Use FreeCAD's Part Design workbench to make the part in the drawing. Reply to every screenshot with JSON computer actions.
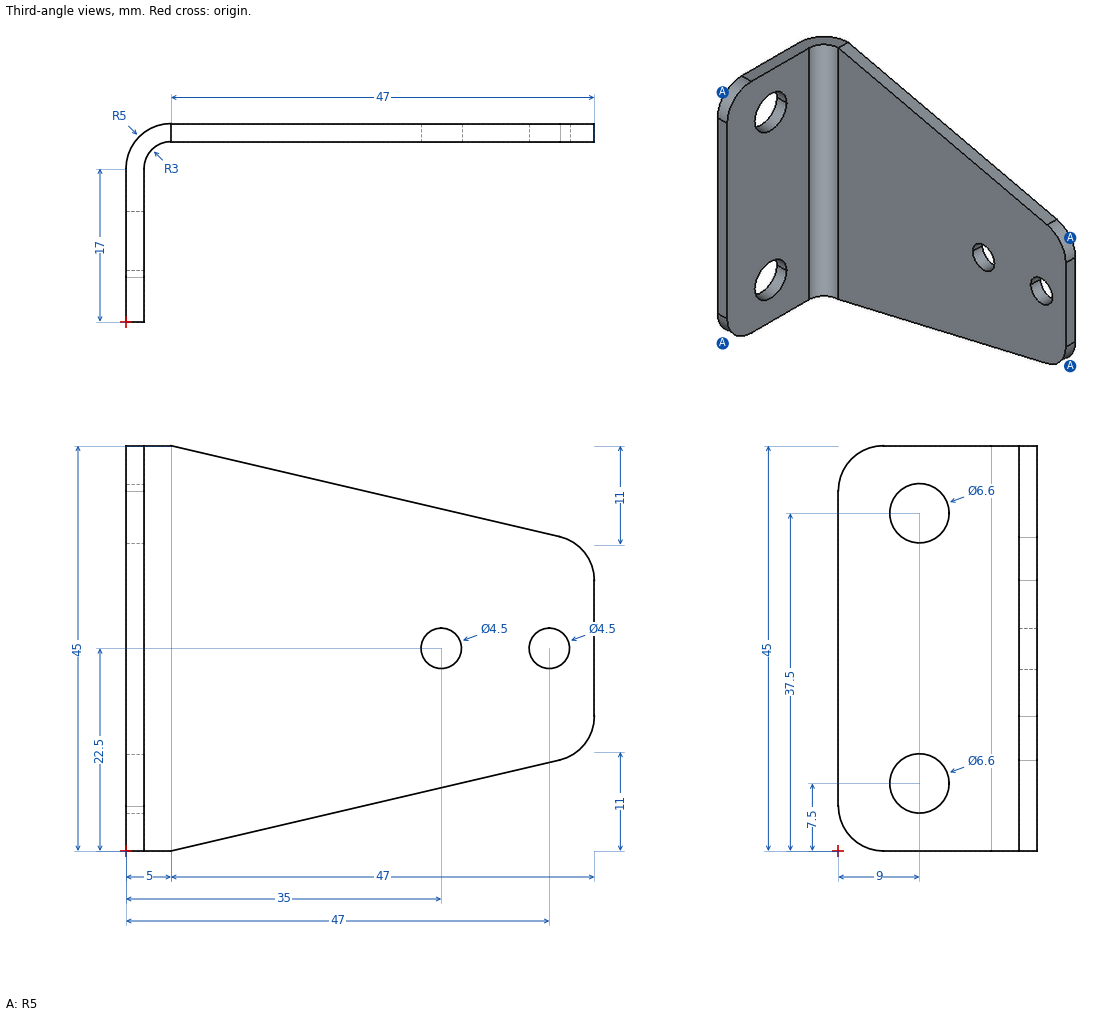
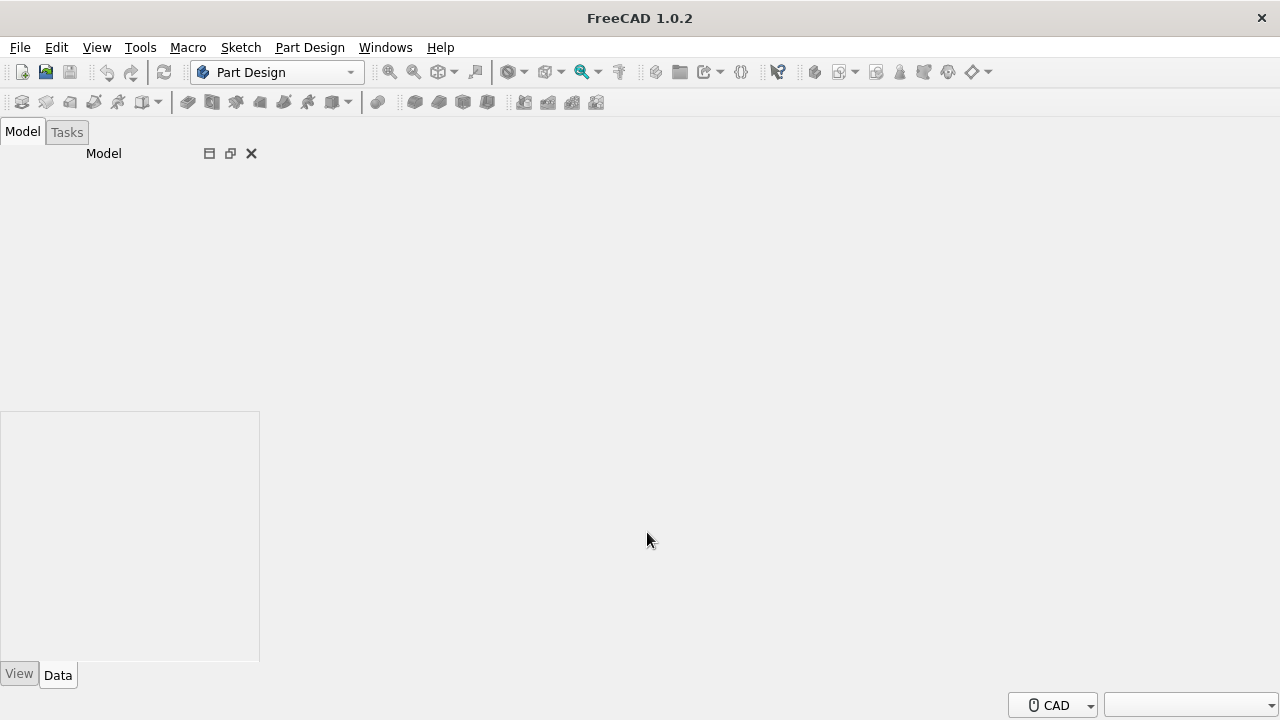
{"action": "key", "text": "ctrl+n"}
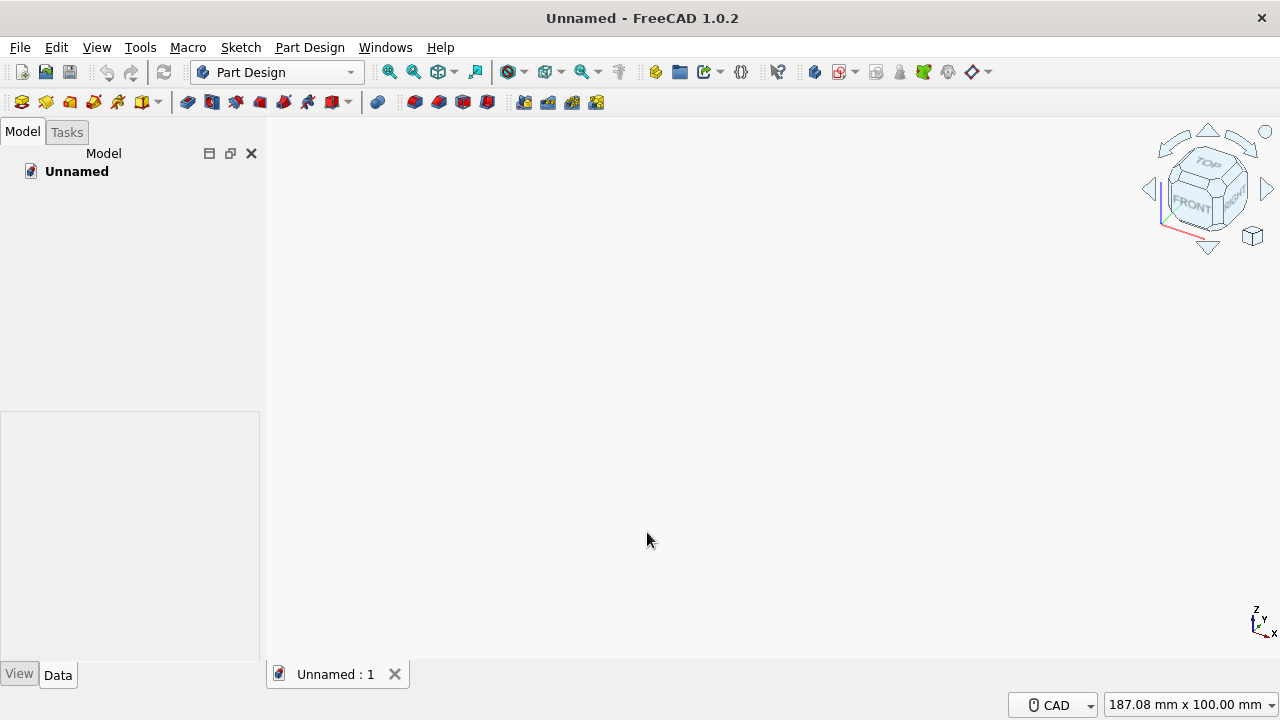
{"action": "left_click", "coordinate": [840, 72]}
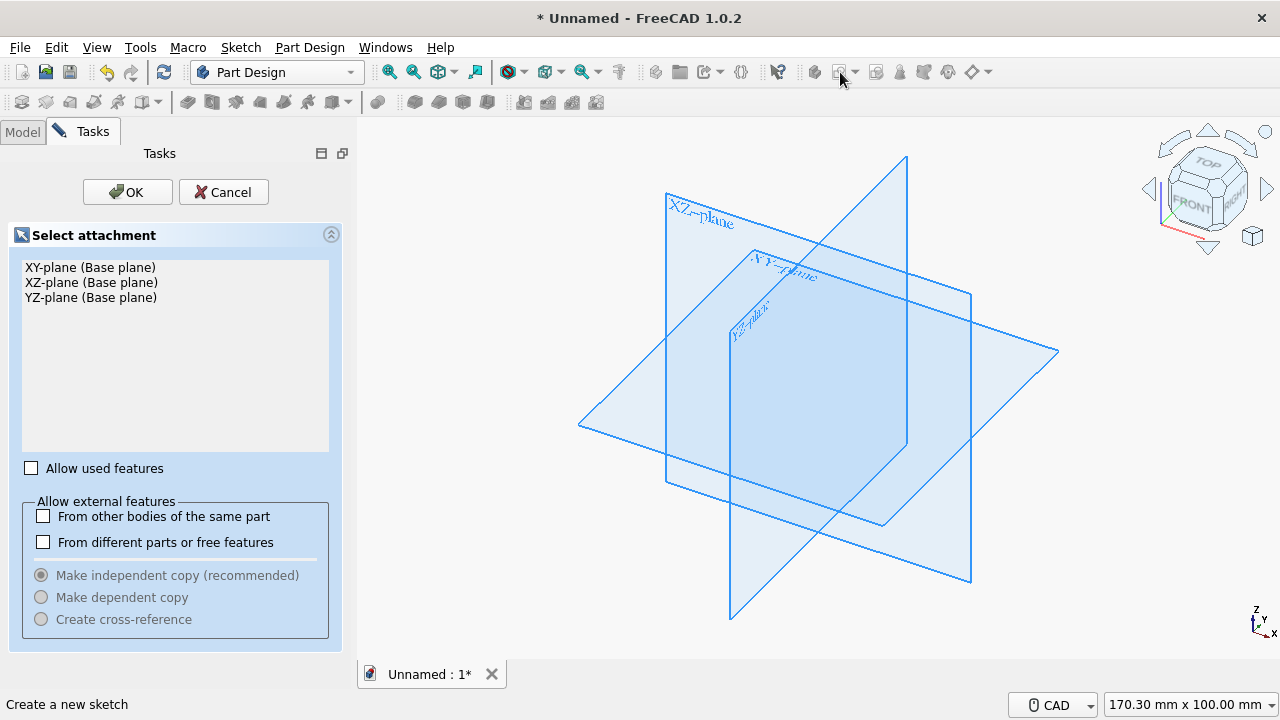
{"action": "left_click", "coordinate": [82, 268]}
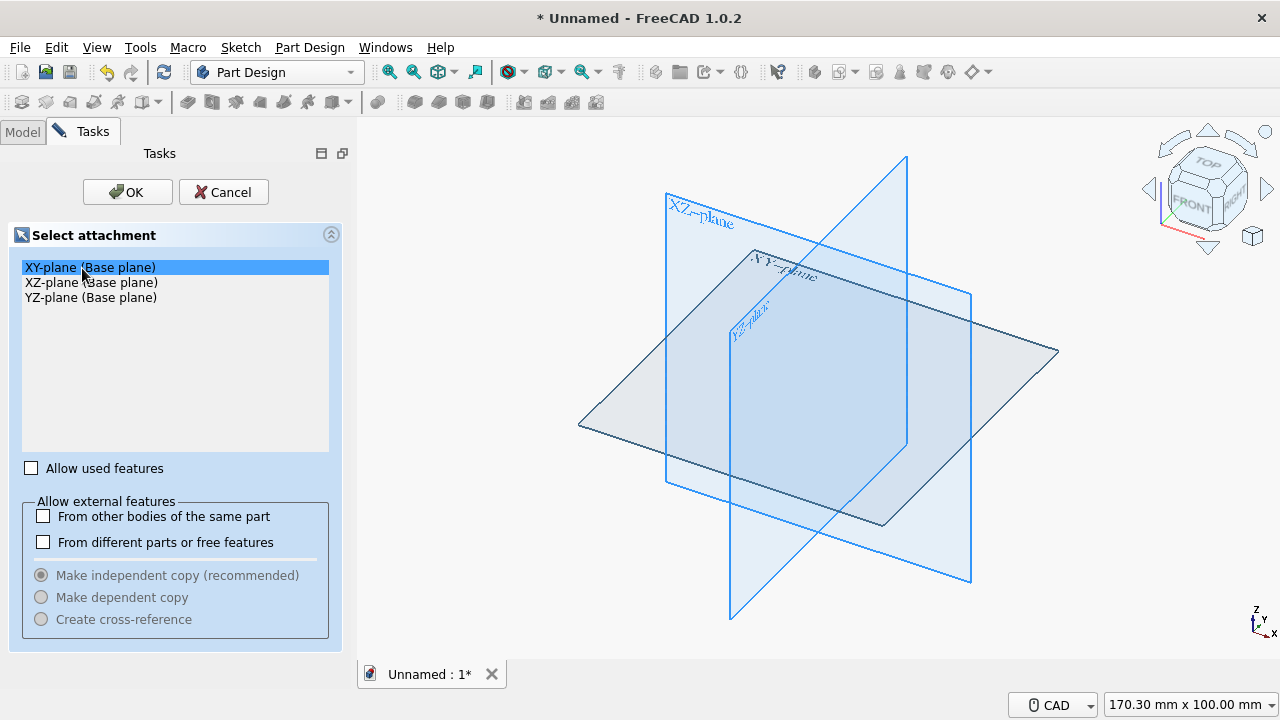
{"action": "left_click", "coordinate": [128, 192]}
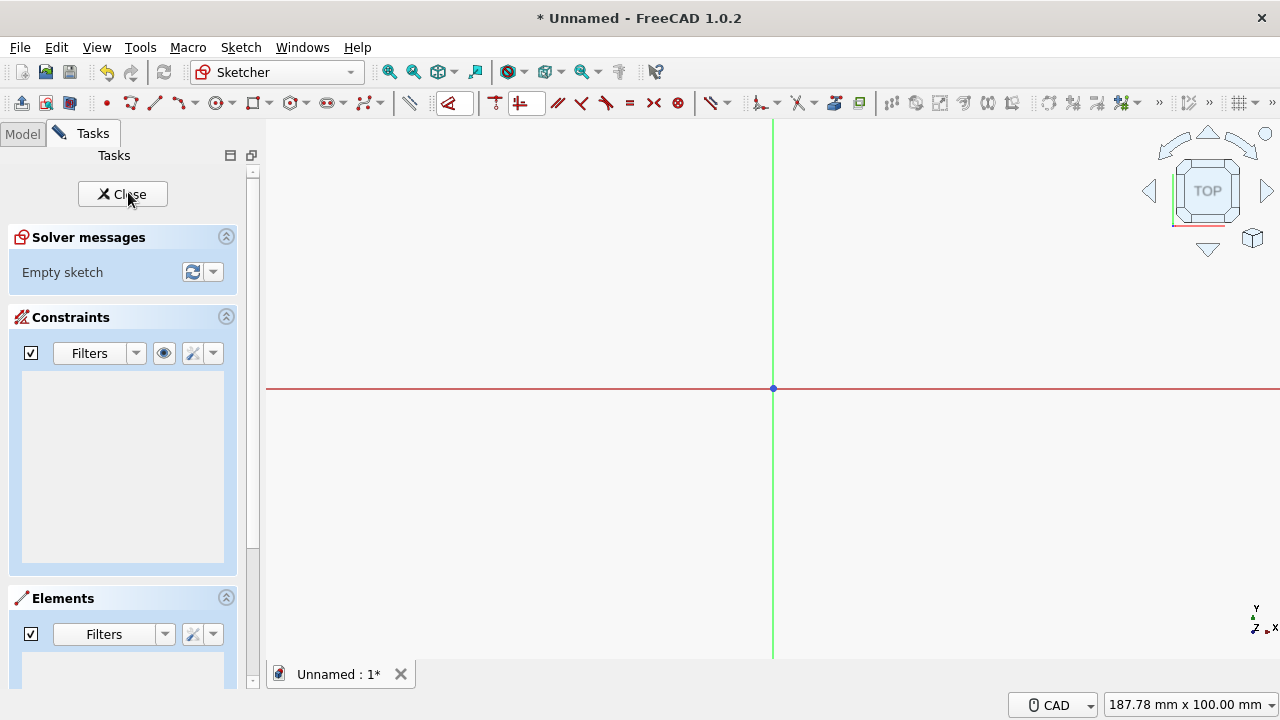
{"action": "scroll", "coordinate": [1084, 281], "scroll_direction": "up", "scroll_amount": 4}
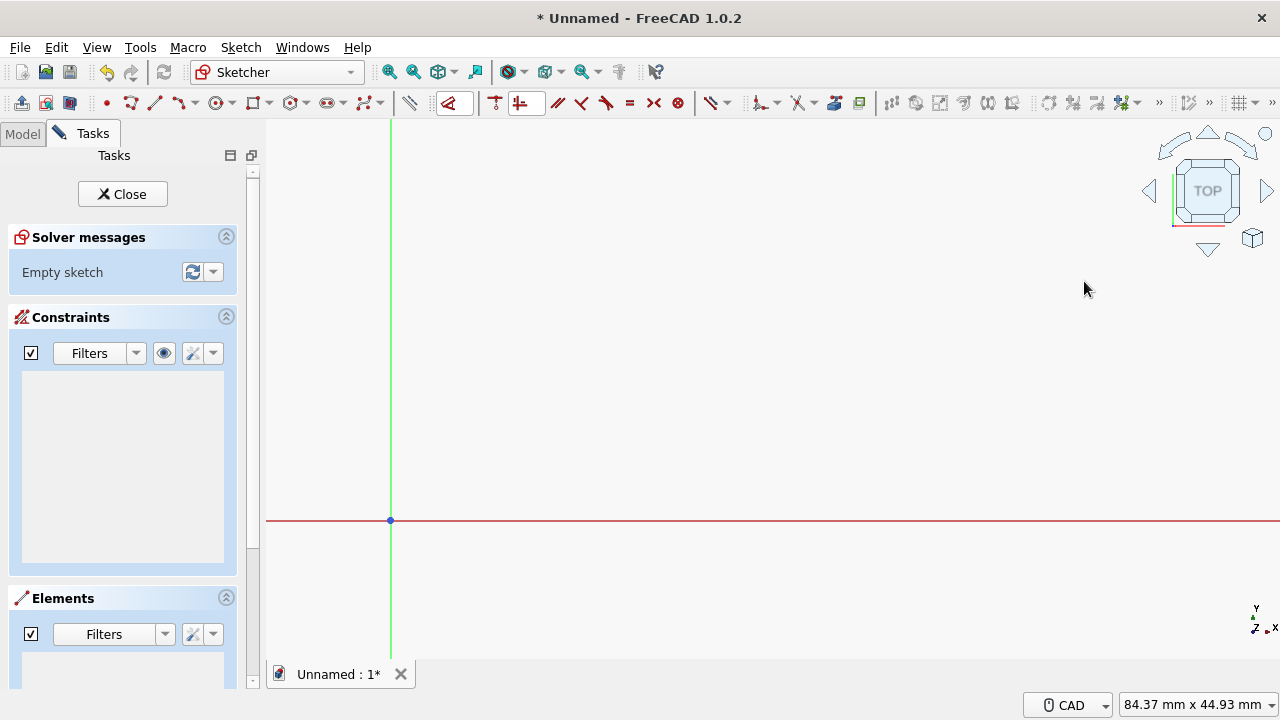
{"action": "left_click", "coordinate": [132, 104]}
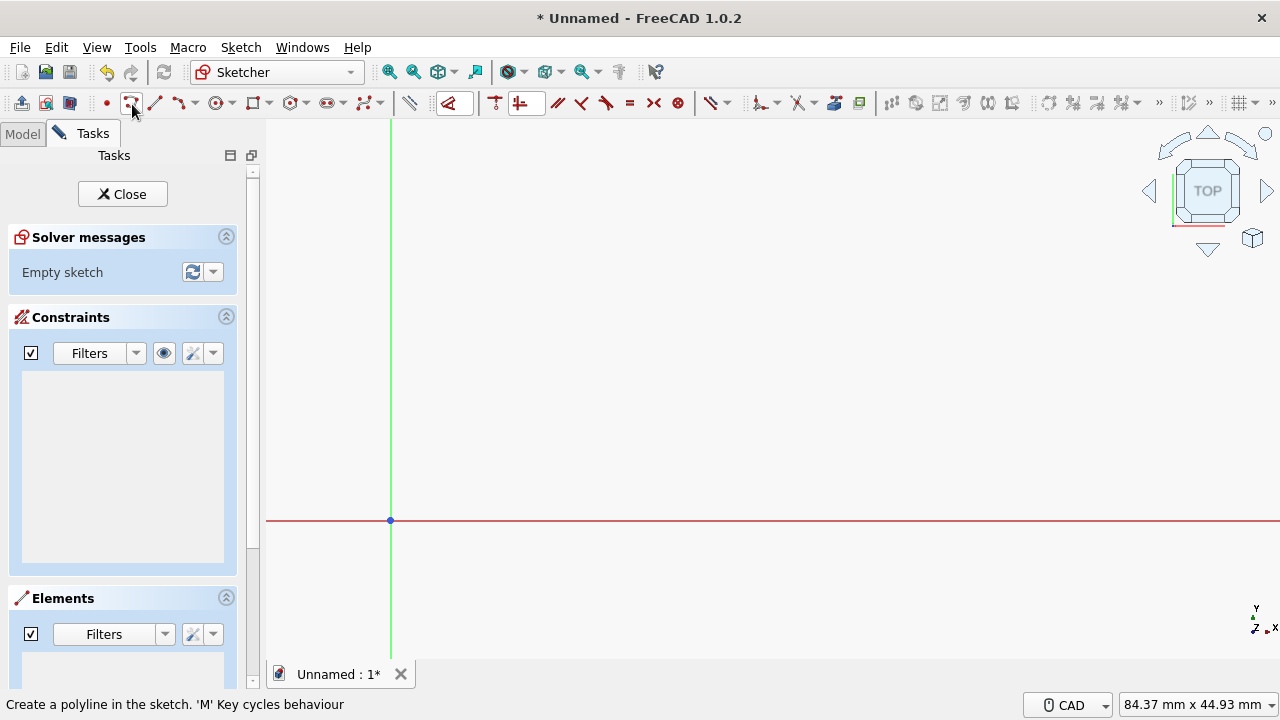
{"action": "left_click", "coordinate": [391, 317]}
{"action": "left_click", "coordinate": [391, 521]}
{"action": "left_click", "coordinate": [415, 512]}
{"action": "left_click", "coordinate": [415, 317]}
{"action": "right_click", "coordinate": [415, 317]}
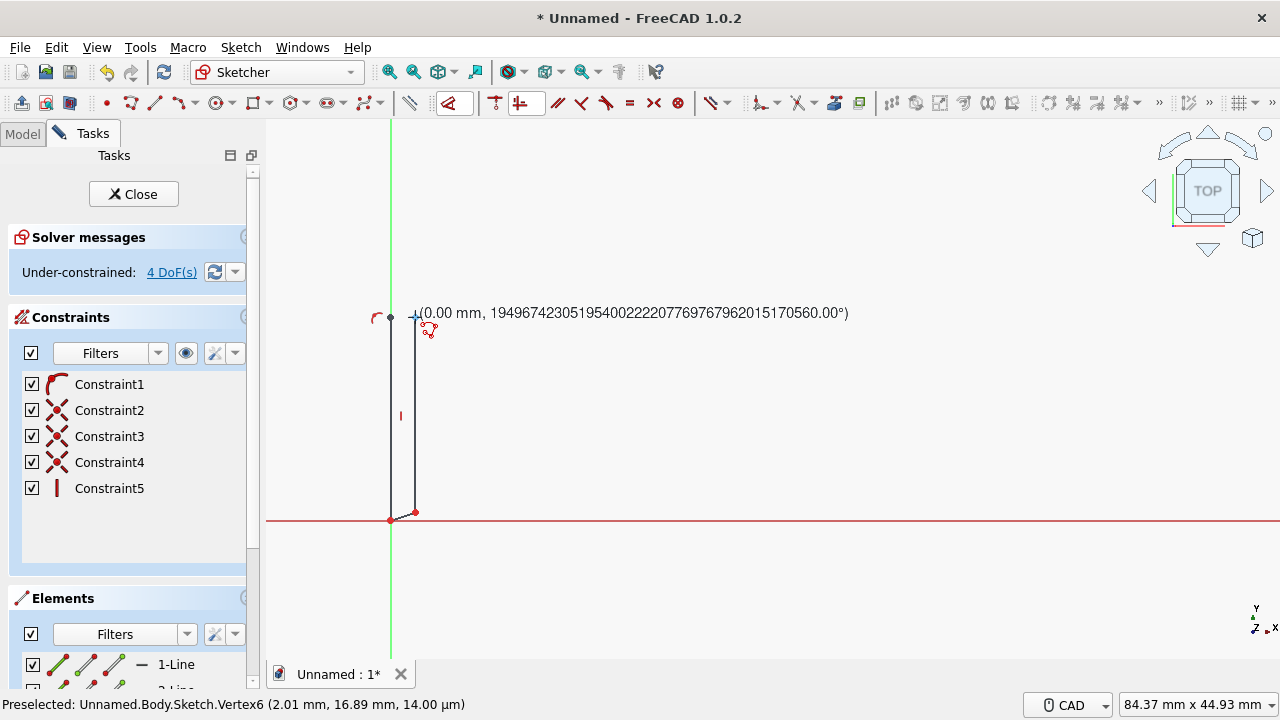
{"action": "left_click", "coordinate": [451, 281]}
{"action": "left_click", "coordinate": [1016, 281]}
{"action": "left_click", "coordinate": [1016, 257]}
{"action": "left_click", "coordinate": [451, 257]}
{"action": "right_click", "coordinate": [451, 257]}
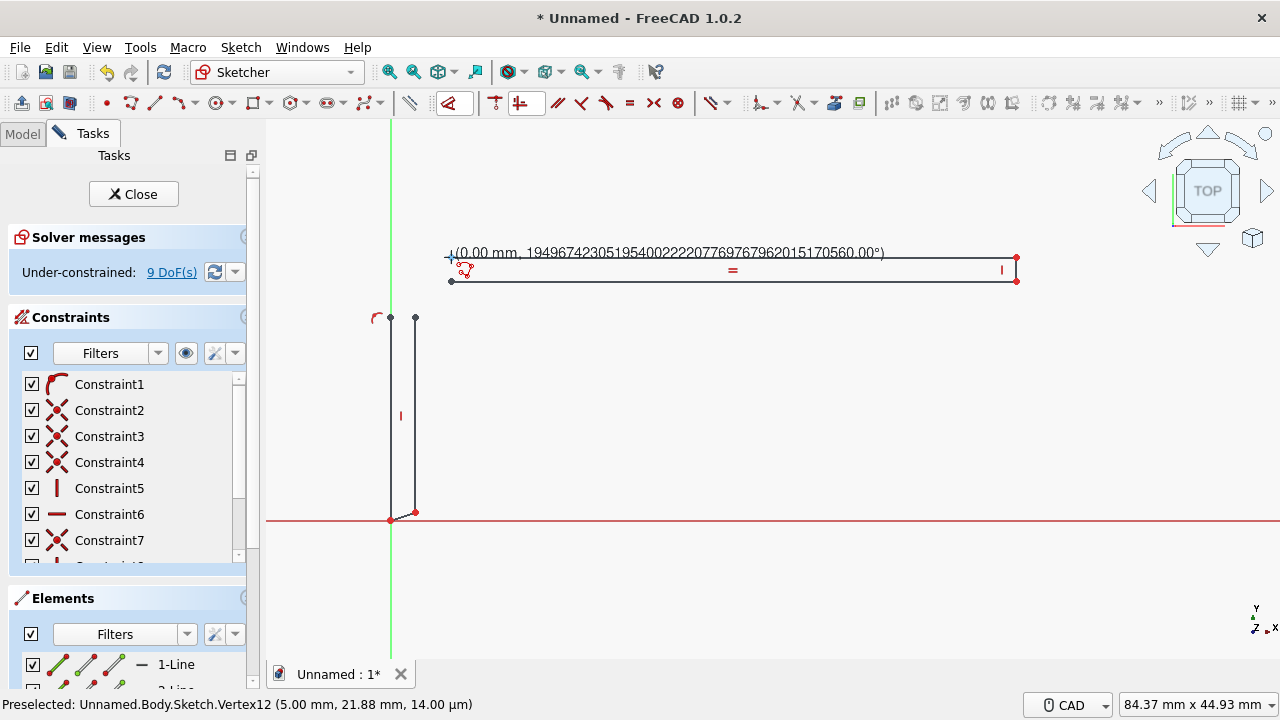
{"action": "key", "text": "g 3 a"}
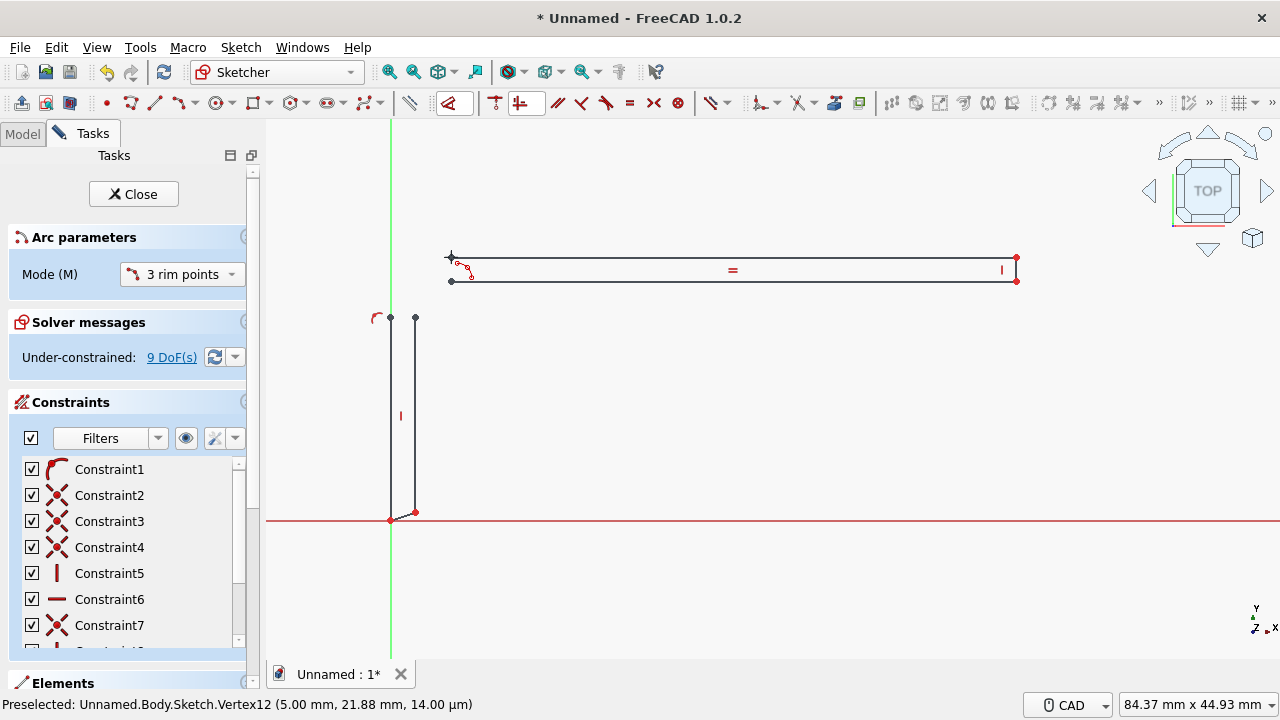
{"action": "left_click", "coordinate": [415, 318]}
{"action": "left_click", "coordinate": [451, 282]}